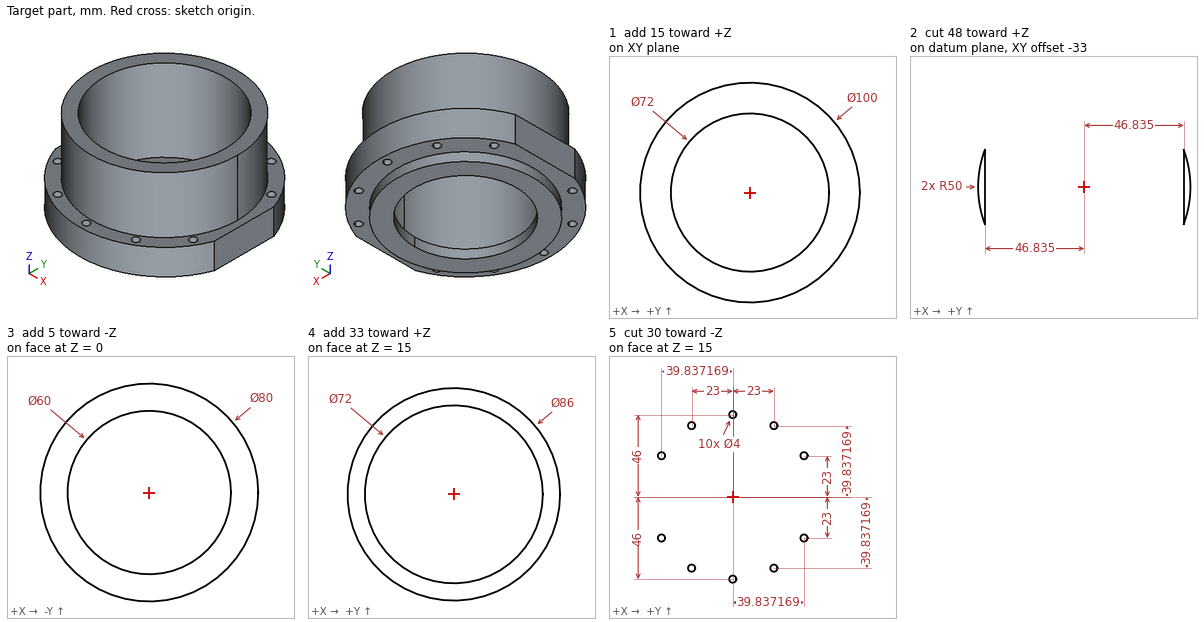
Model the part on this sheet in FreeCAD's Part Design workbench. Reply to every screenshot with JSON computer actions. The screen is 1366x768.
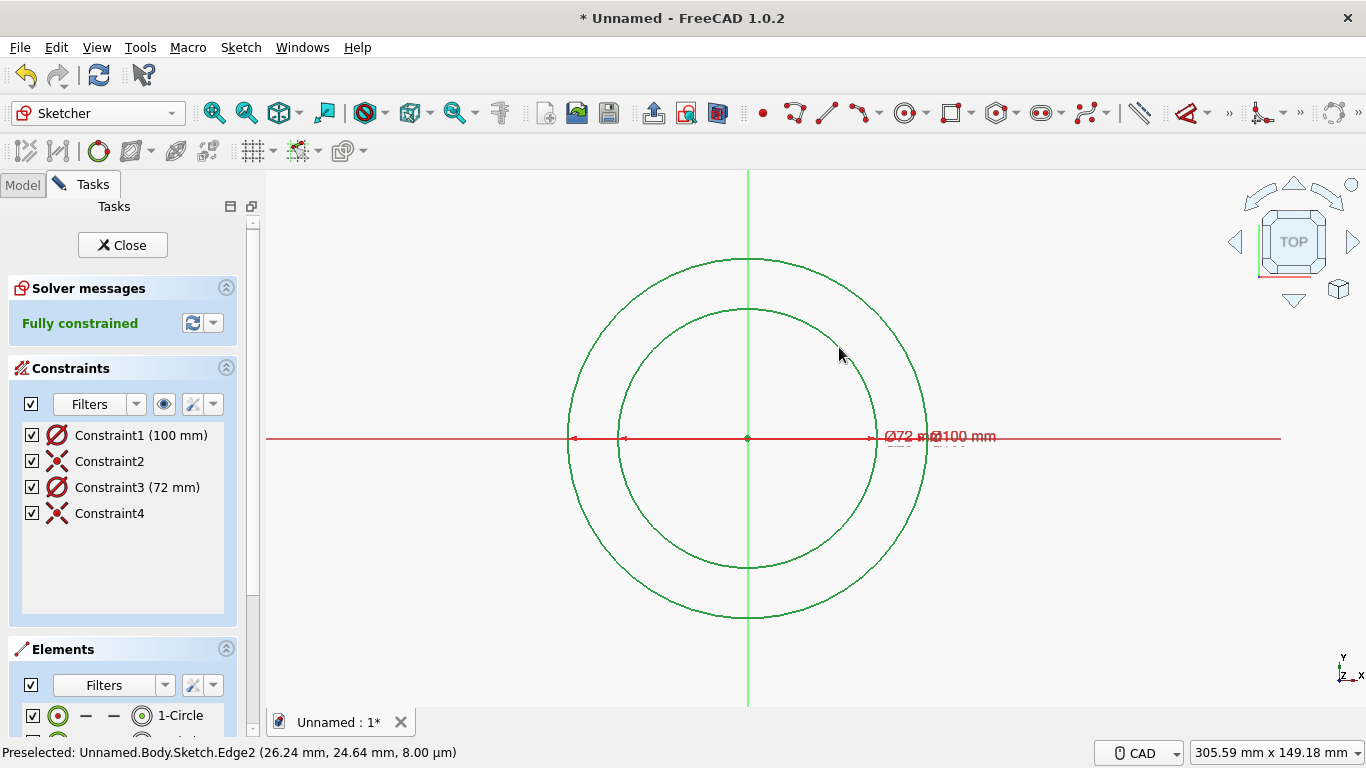
{"action": "left_click", "coordinate": [123, 245]}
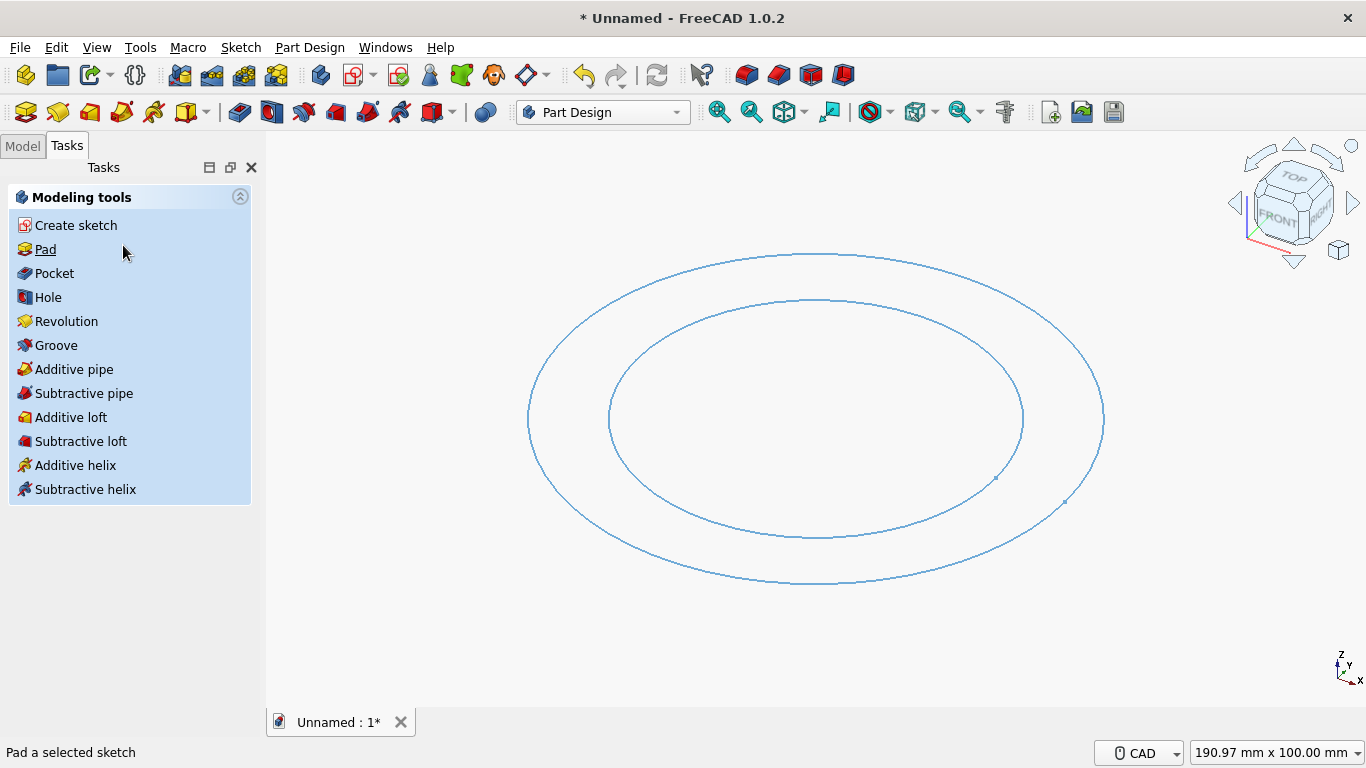
{"action": "left_click", "coordinate": [26, 112]}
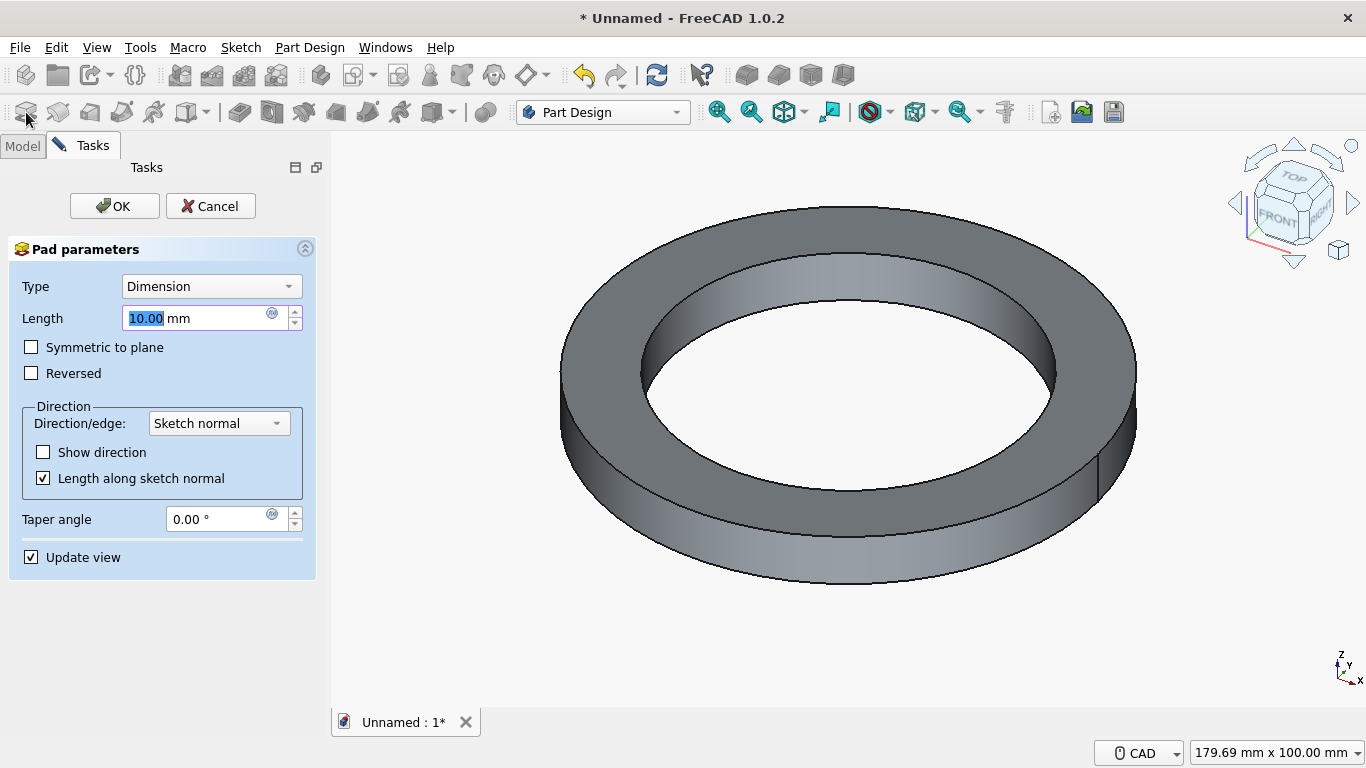
{"action": "type", "text": "15"}
{"action": "key", "text": "Tab"}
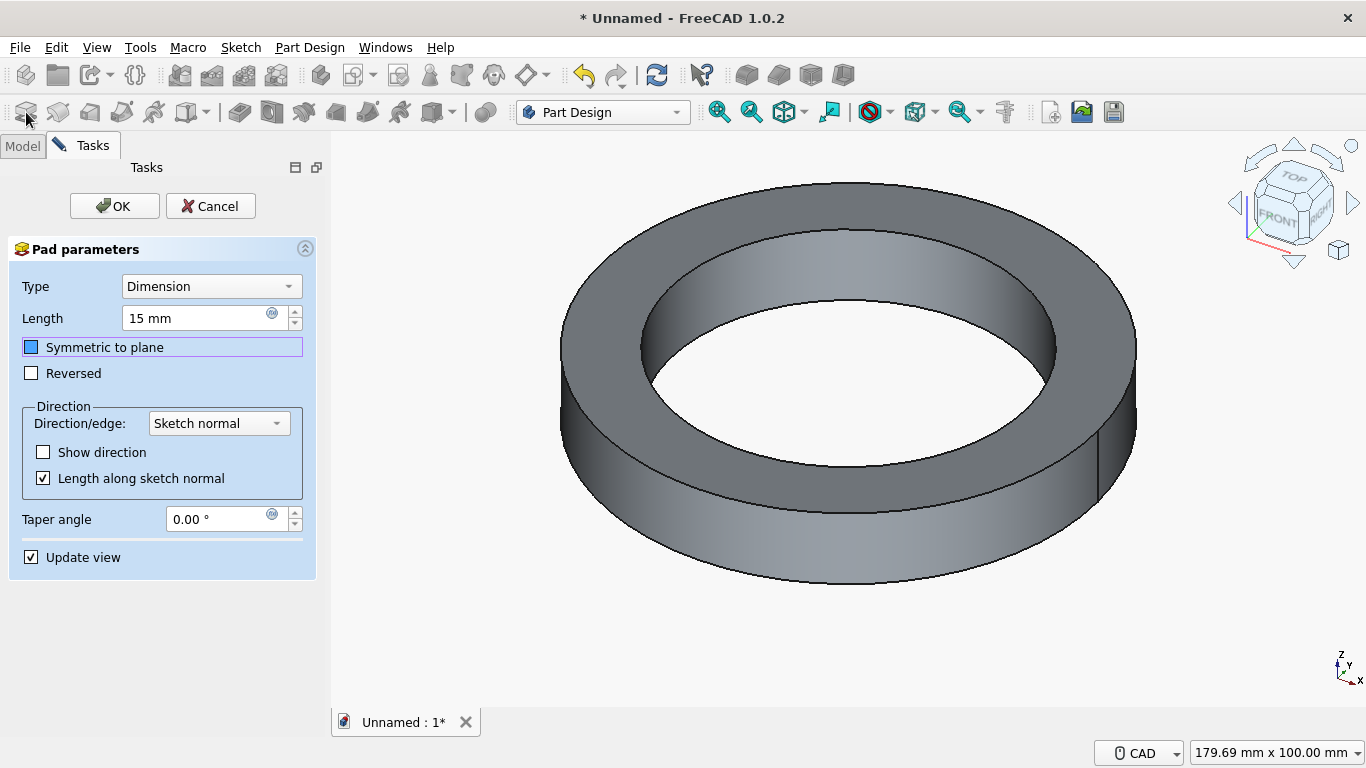
{"action": "left_click", "coordinate": [115, 206]}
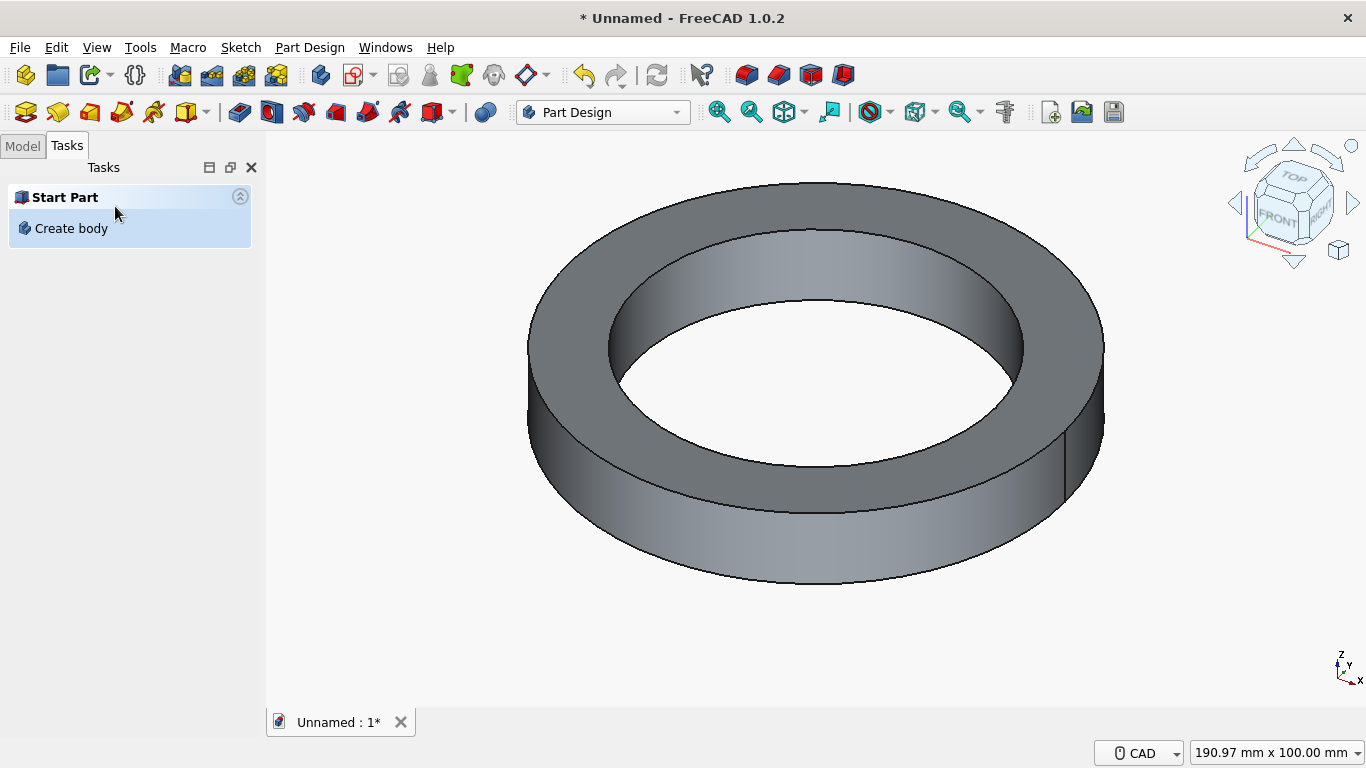
{"action": "left_click", "coordinate": [720, 112]}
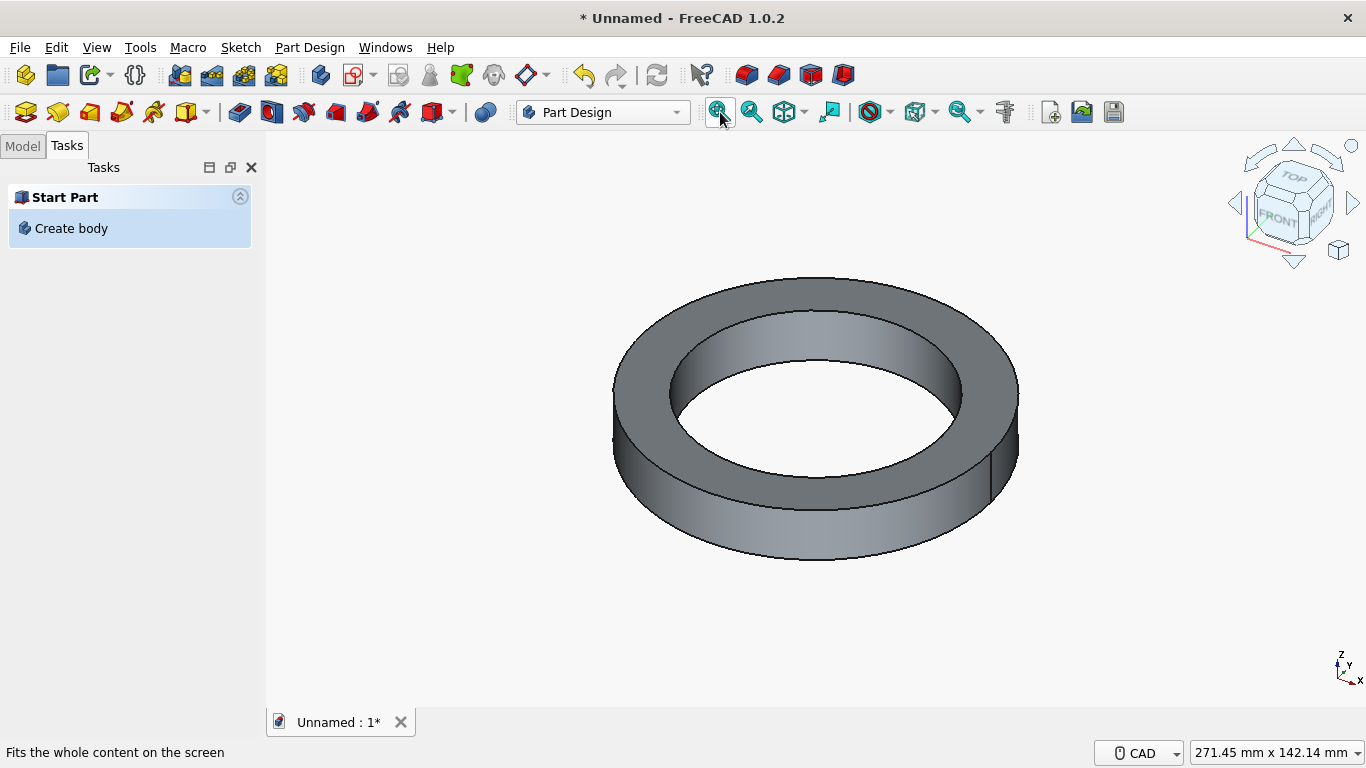
{"action": "left_click", "coordinate": [23, 145]}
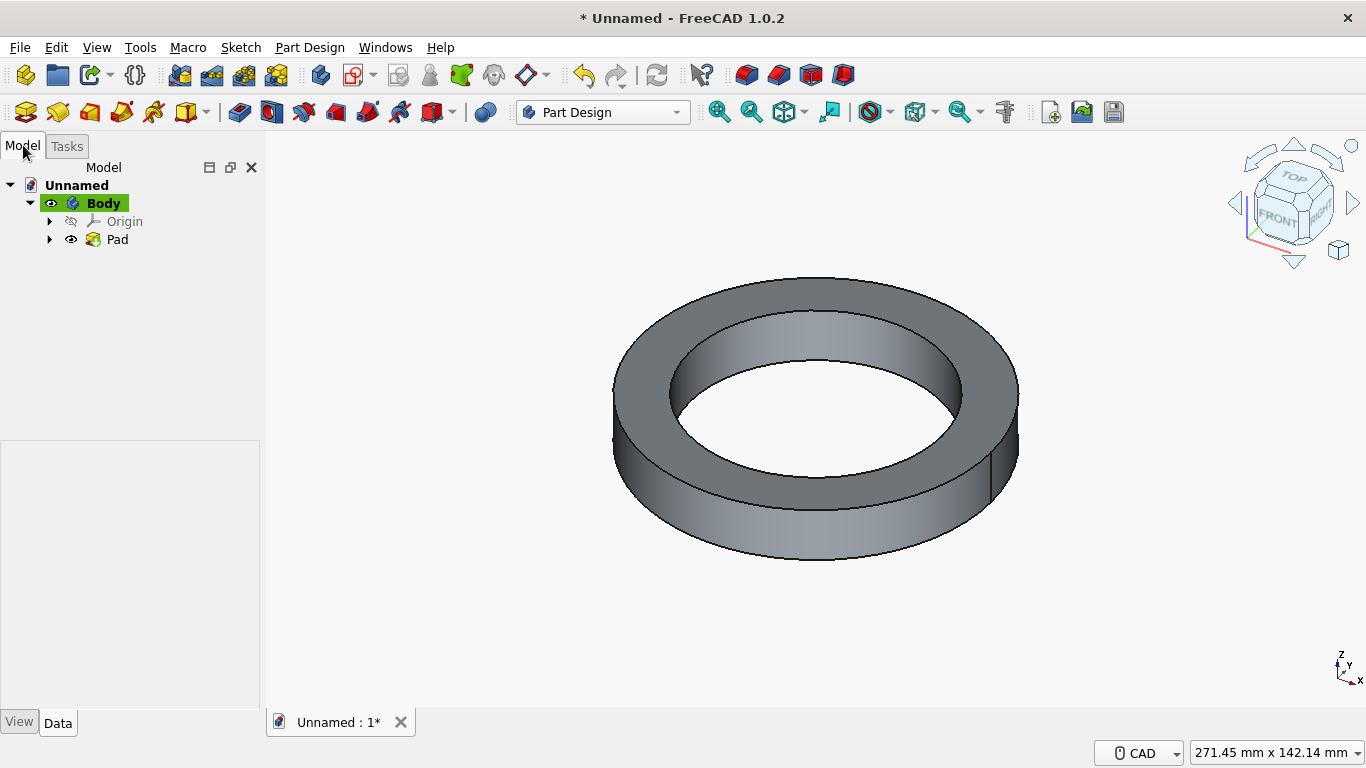
{"action": "left_click", "coordinate": [50, 221]}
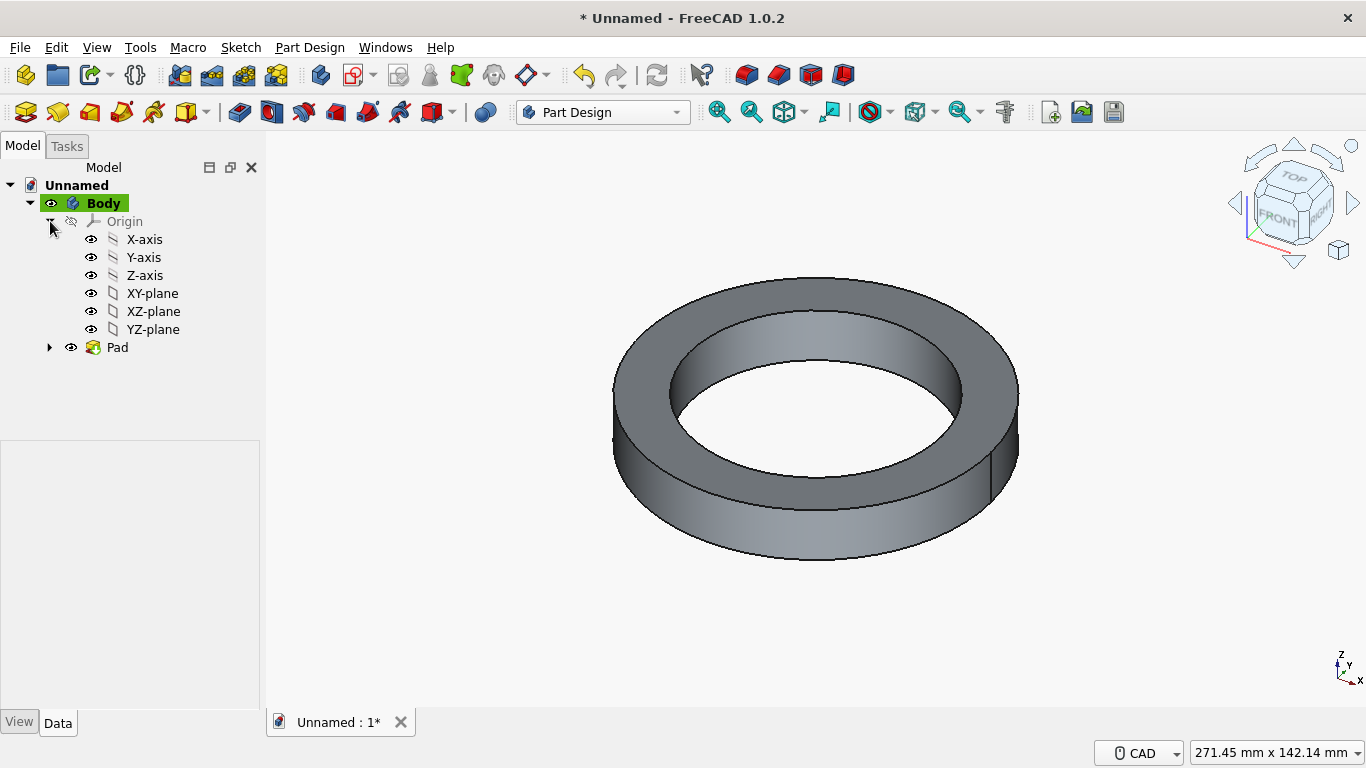
{"action": "left_click", "coordinate": [136, 293]}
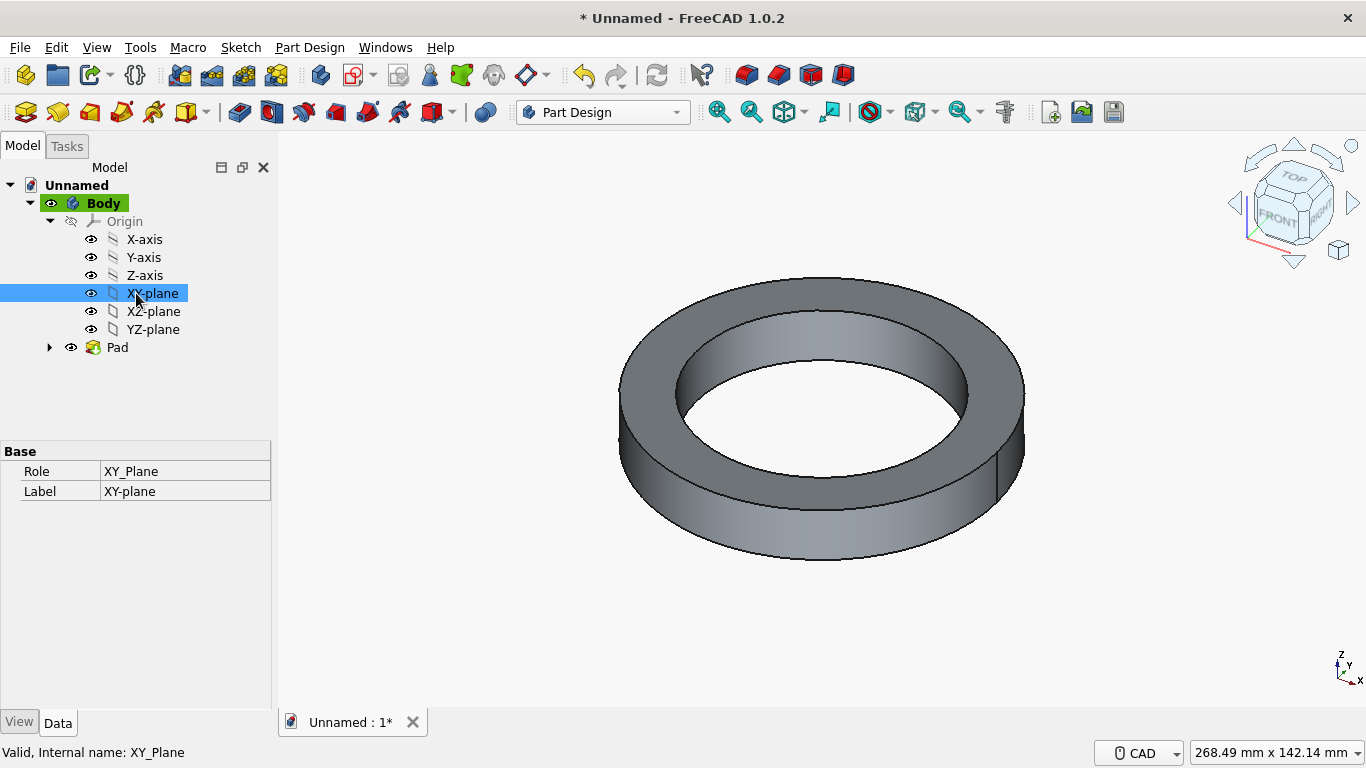
{"action": "left_click", "coordinate": [526, 76]}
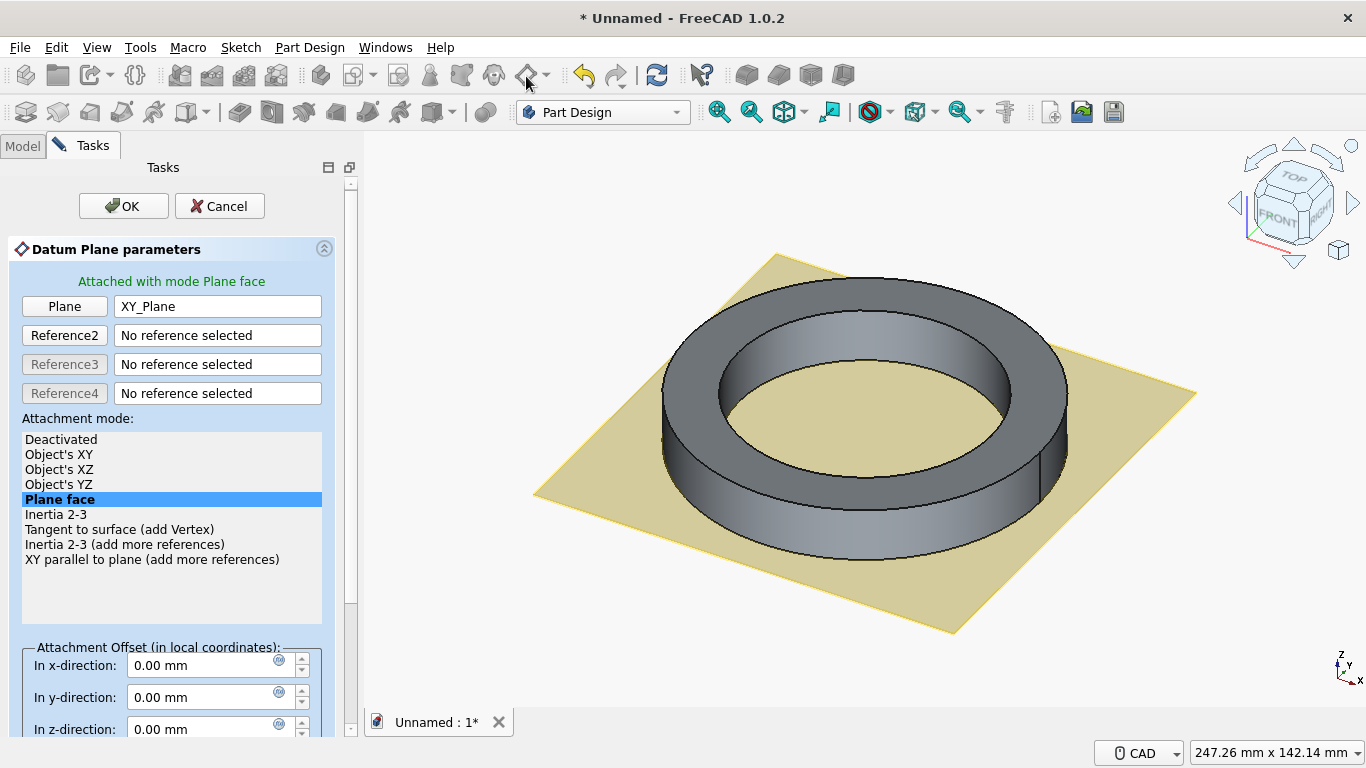
{"action": "scroll", "coordinate": [351, 456], "scroll_direction": "down", "scroll_amount": 2}